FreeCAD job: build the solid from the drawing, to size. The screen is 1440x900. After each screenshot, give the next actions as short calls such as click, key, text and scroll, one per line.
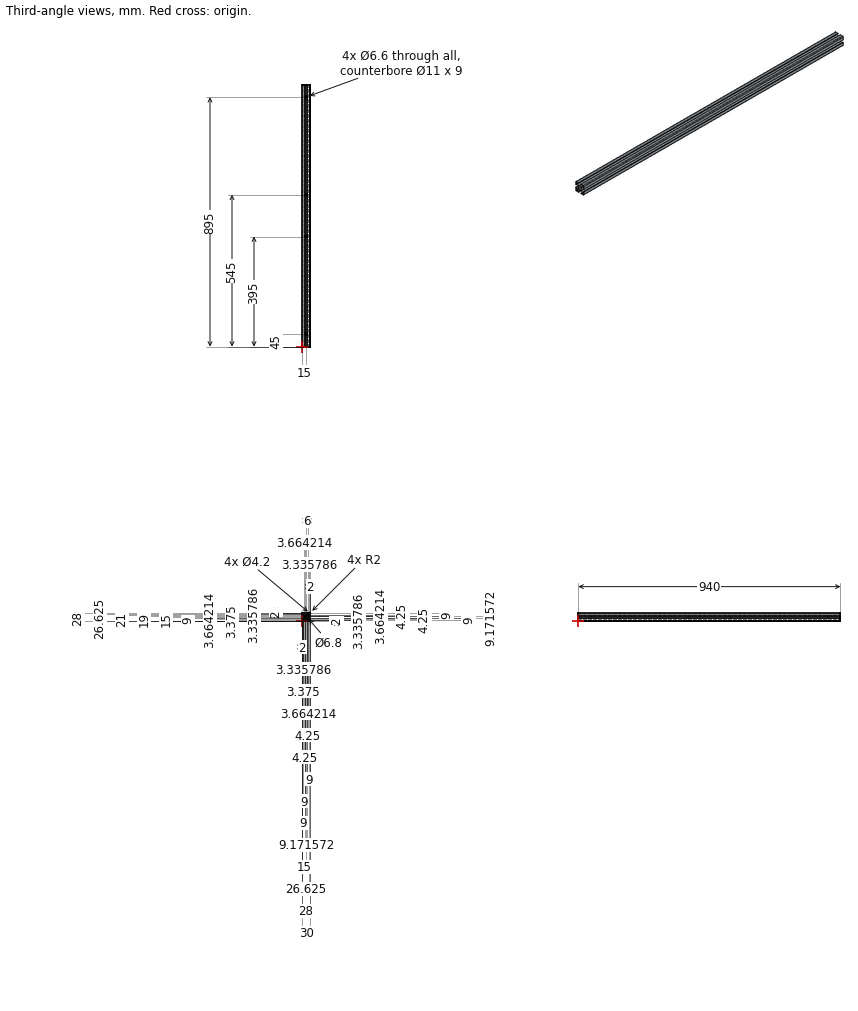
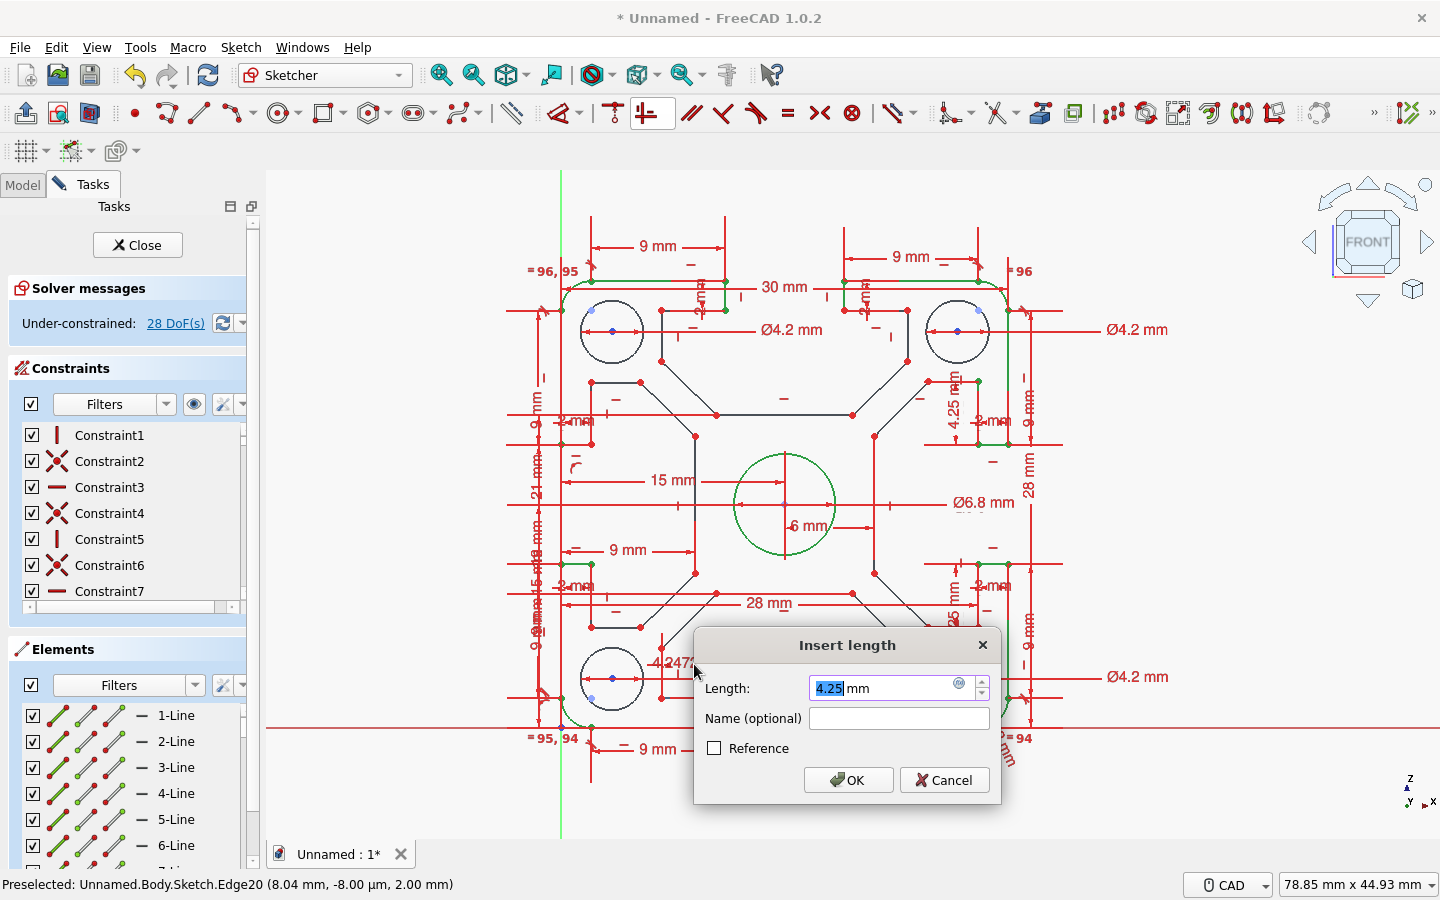
text(4.25)
key(Return)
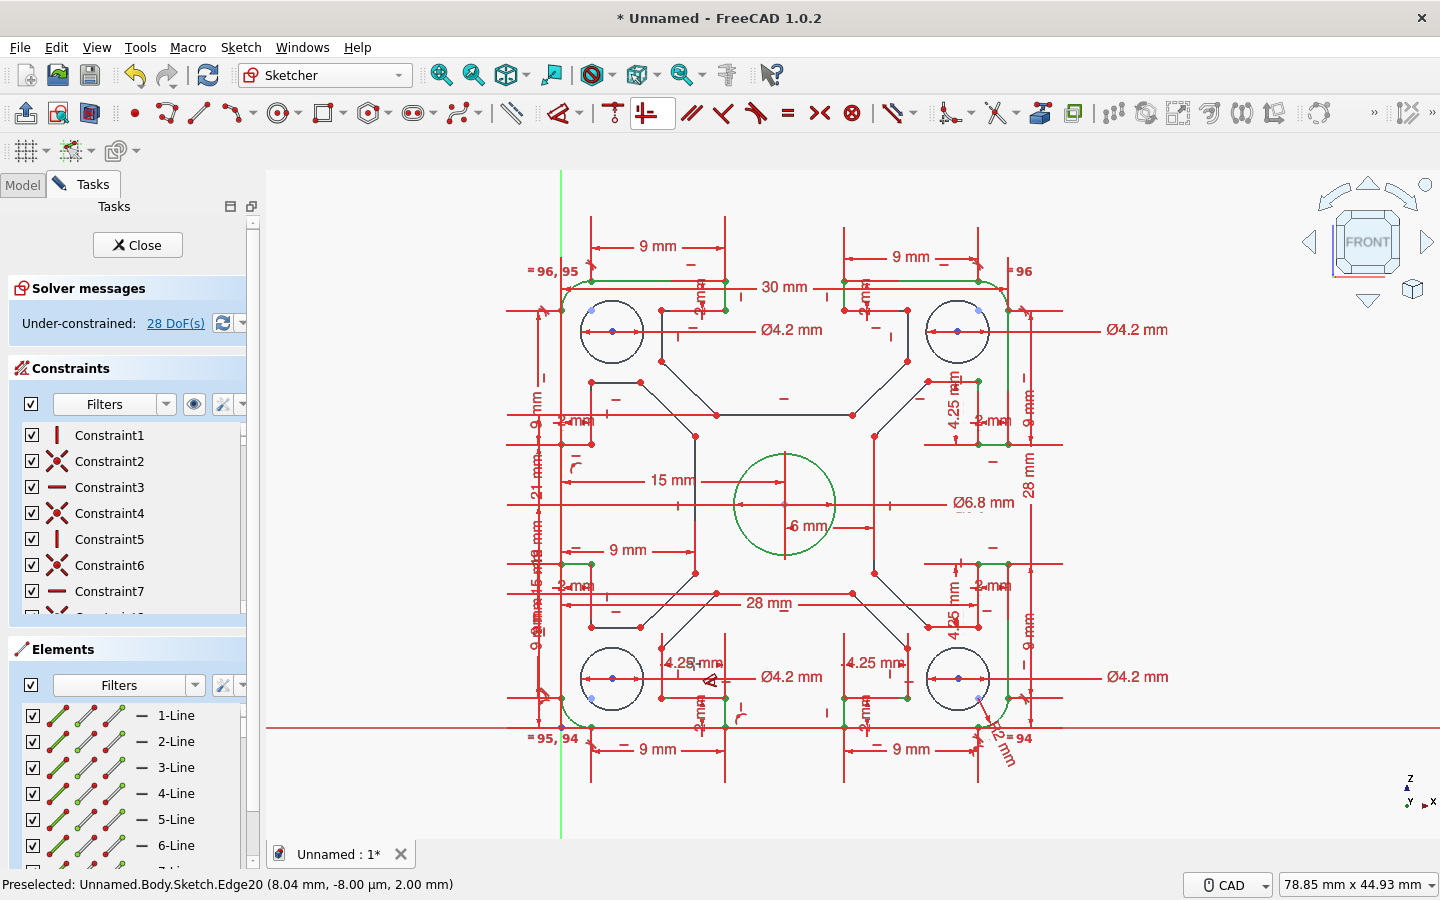
click(591, 583)
click(625, 611)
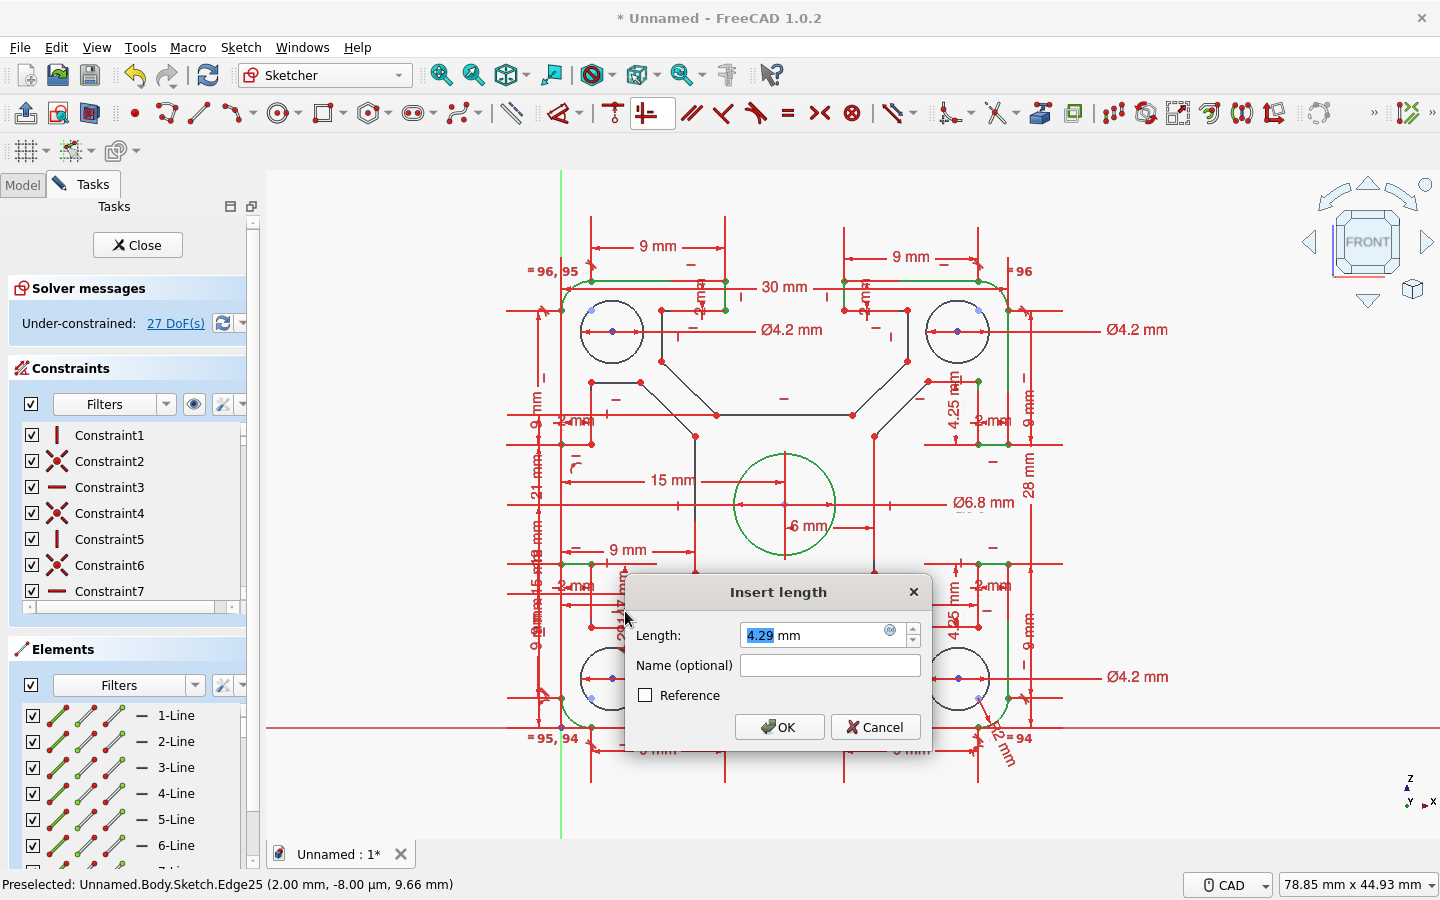
text(4.25)
key(Return)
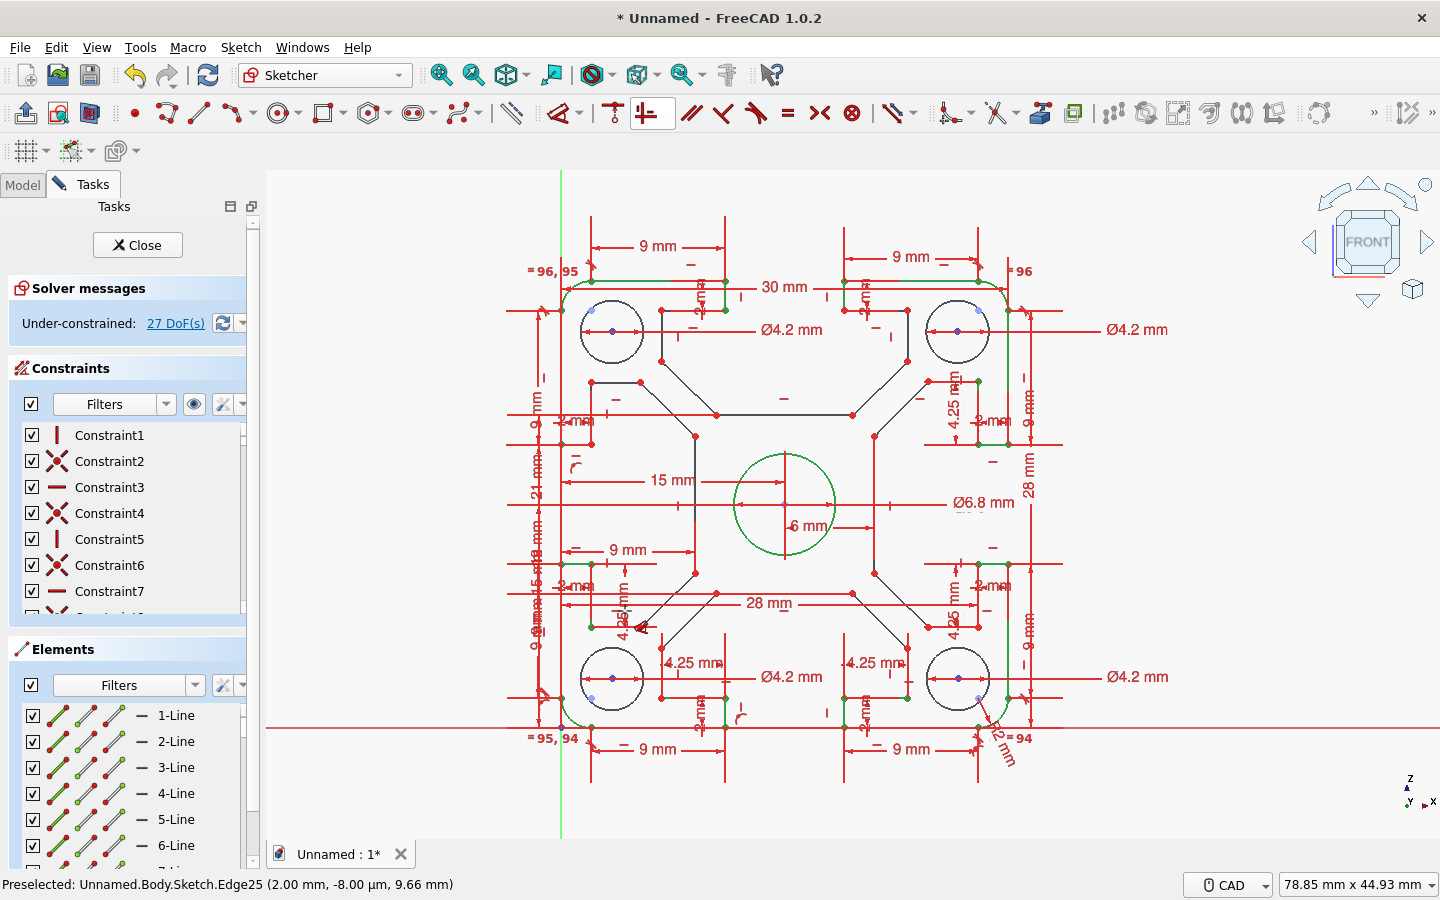
click(591, 402)
click(625, 400)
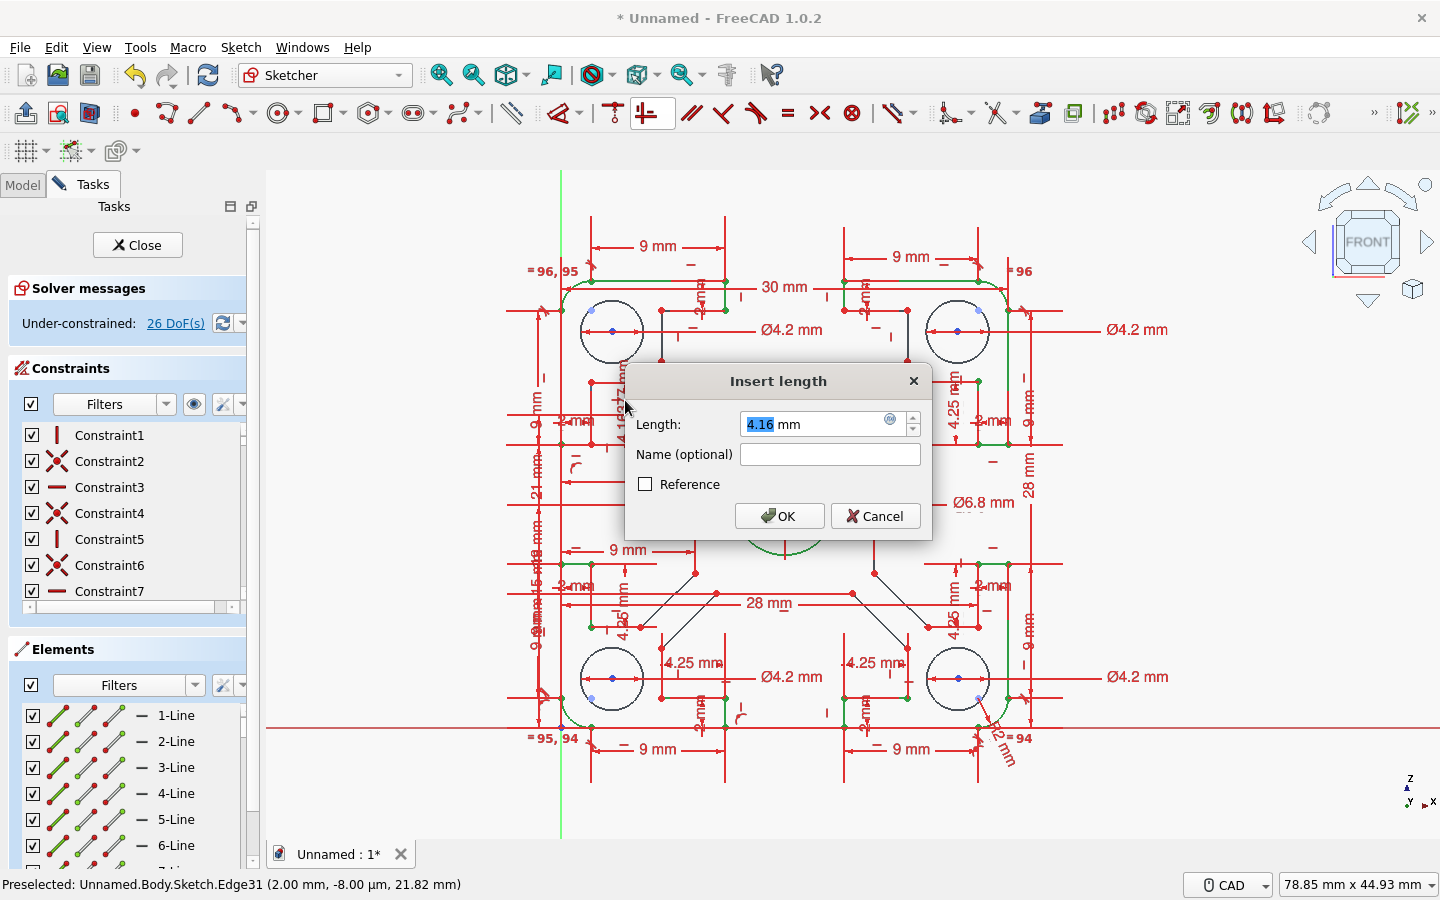
text(4.25)
key(Return)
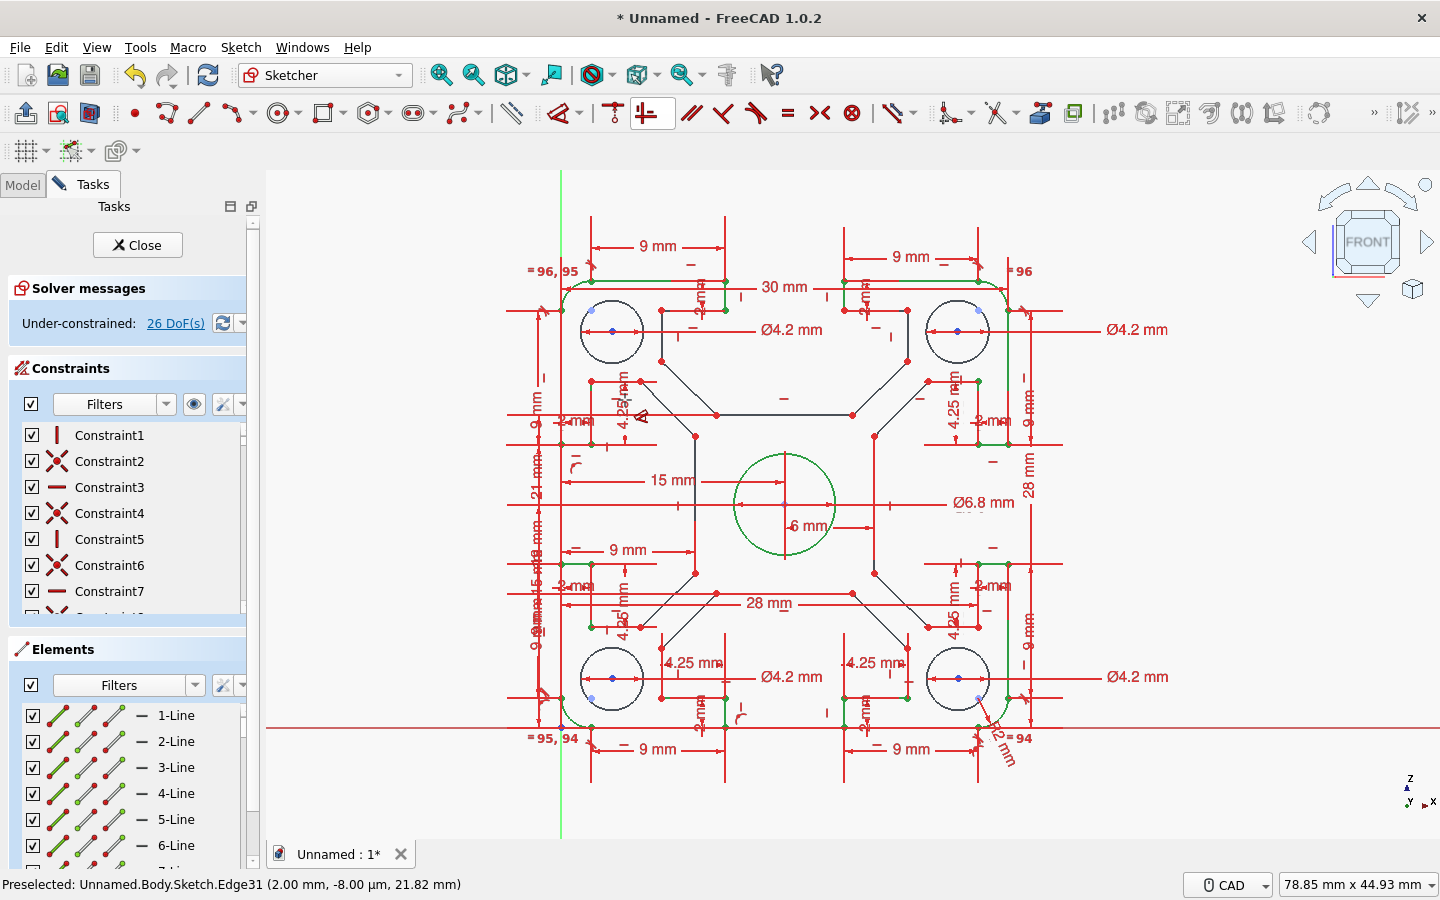
click(706, 311)
click(694, 345)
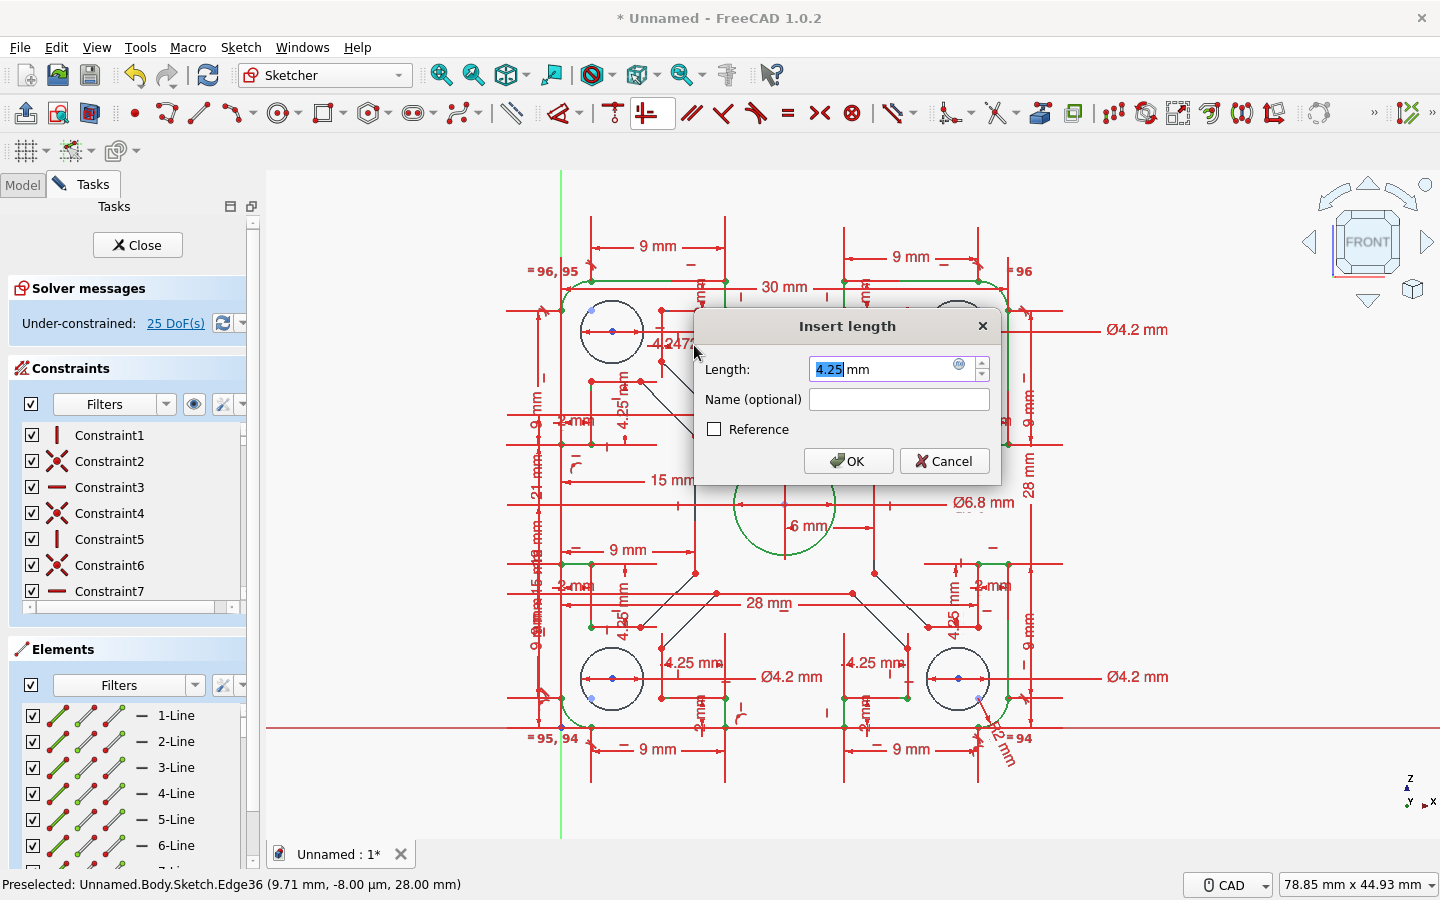
text(4.25)
key(Return)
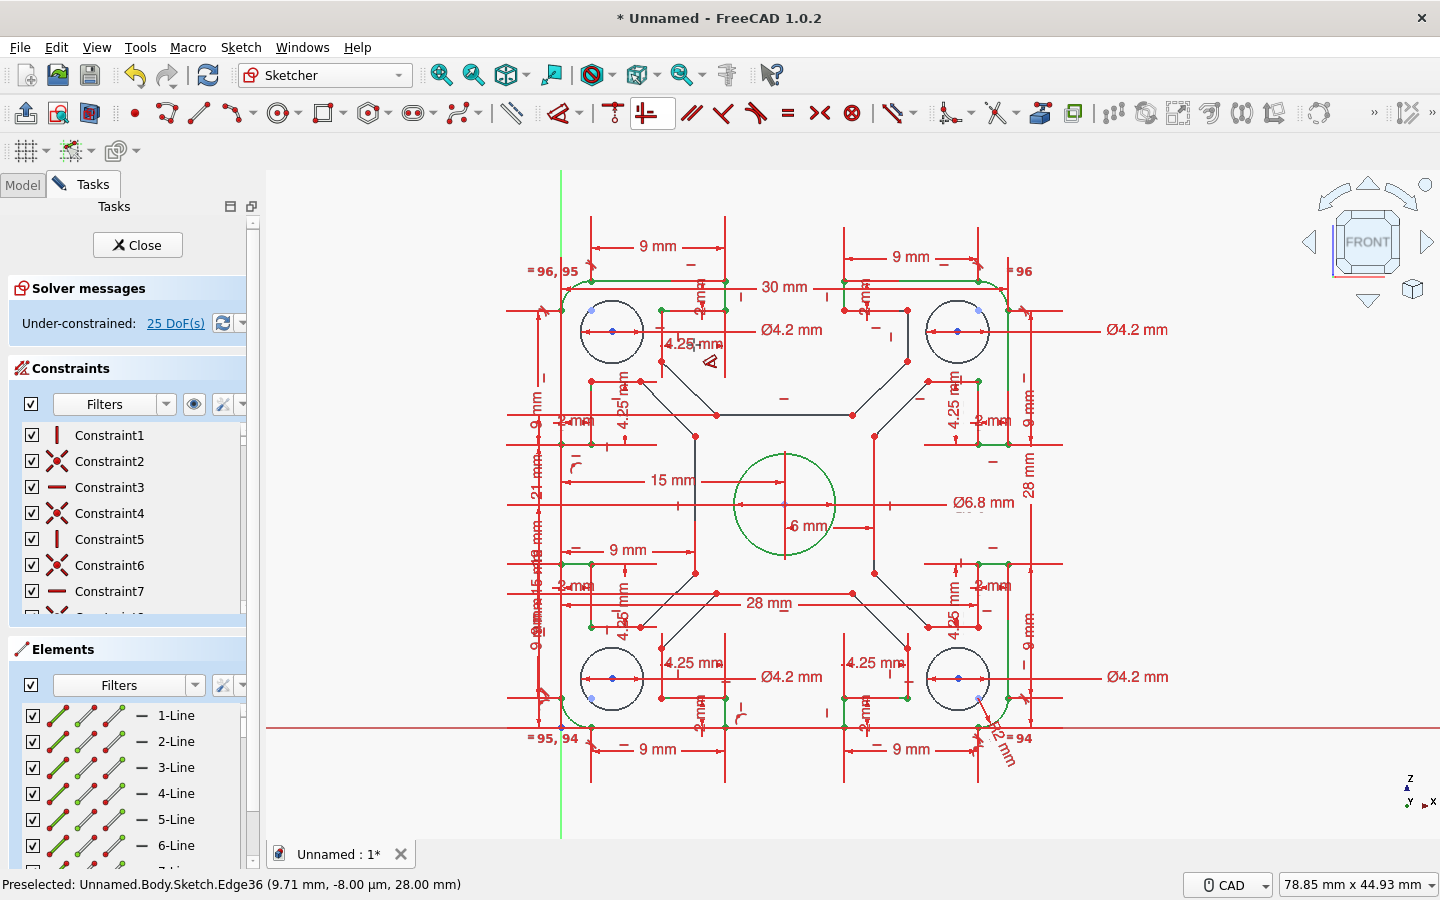
click(889, 311)
click(876, 345)